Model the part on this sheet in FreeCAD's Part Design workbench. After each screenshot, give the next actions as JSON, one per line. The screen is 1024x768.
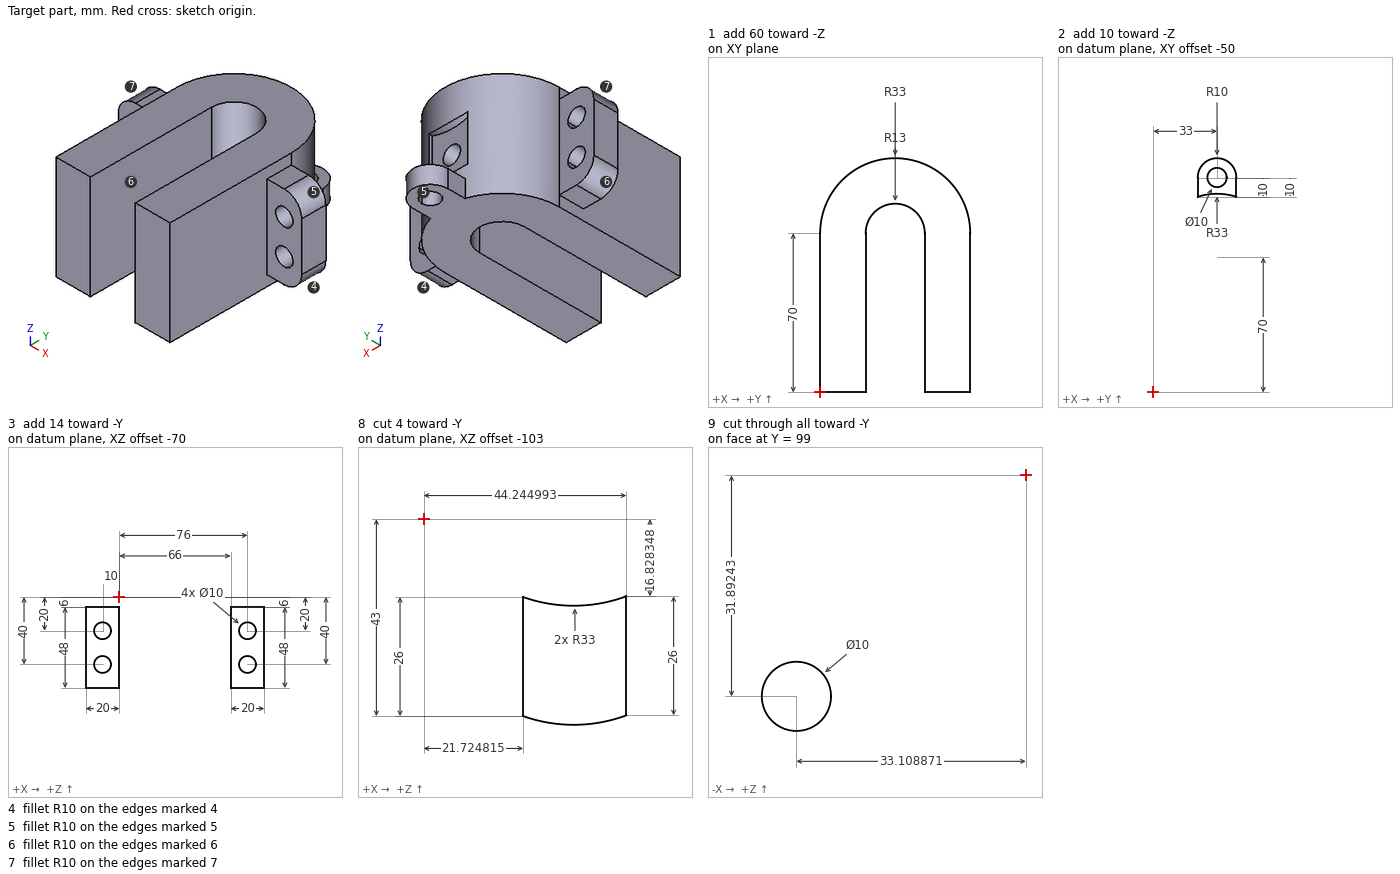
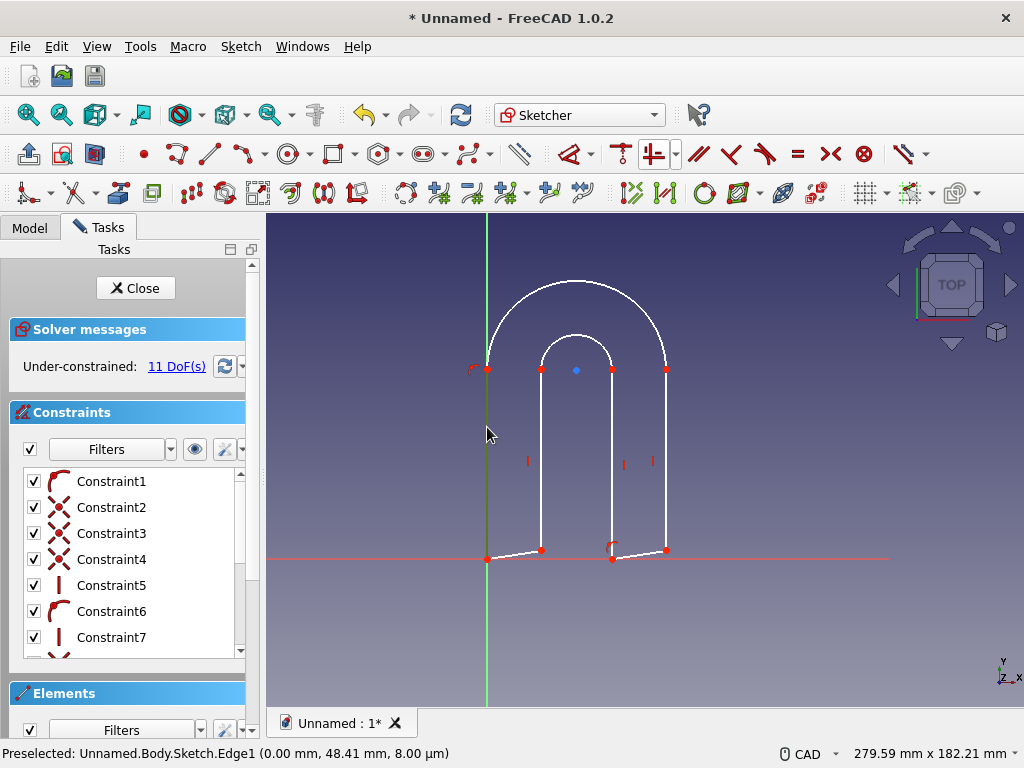
{"action": "left_click", "coordinate": [629, 298]}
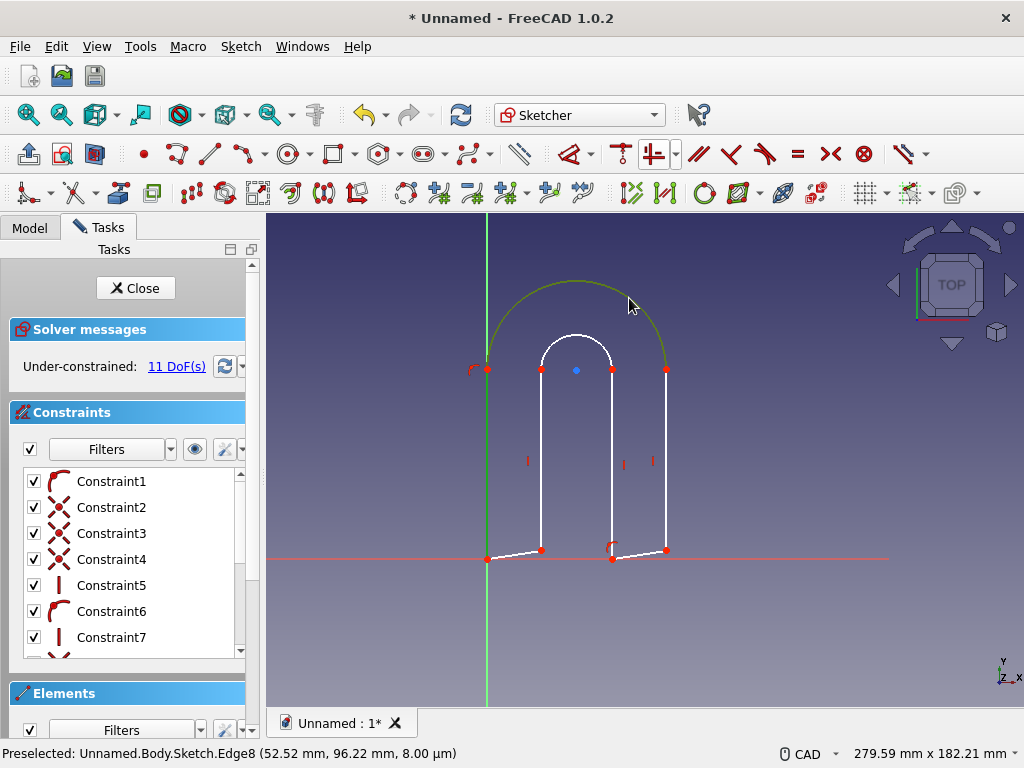
{"action": "key", "text": "t"}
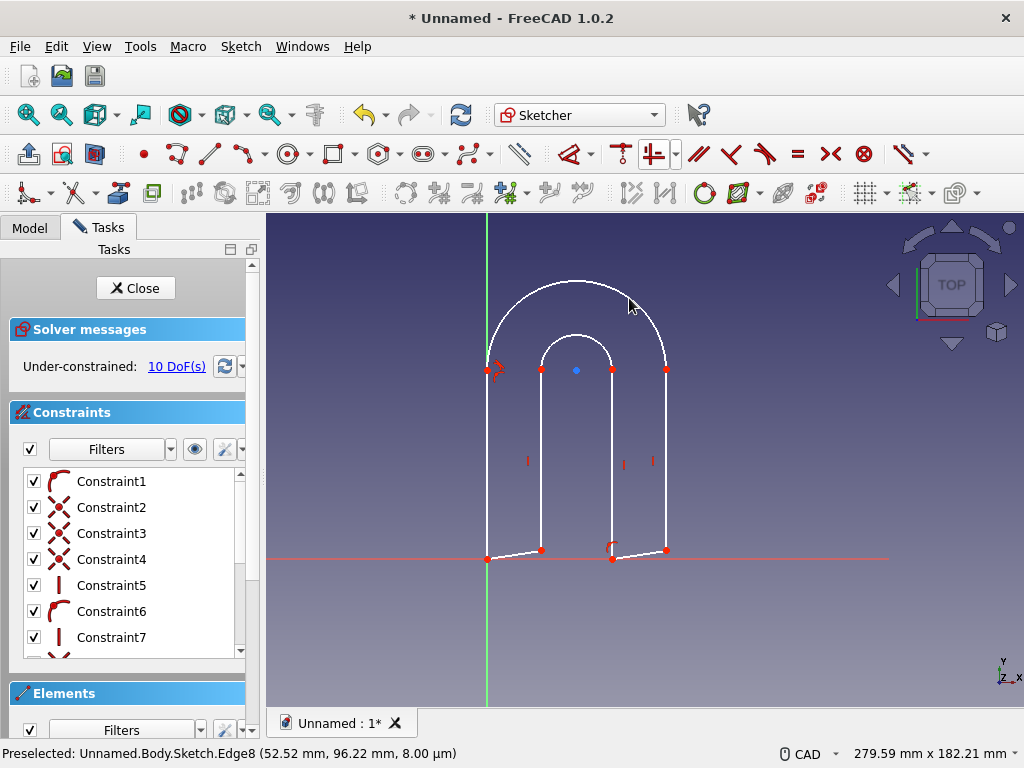
{"action": "left_click", "coordinate": [541, 497]}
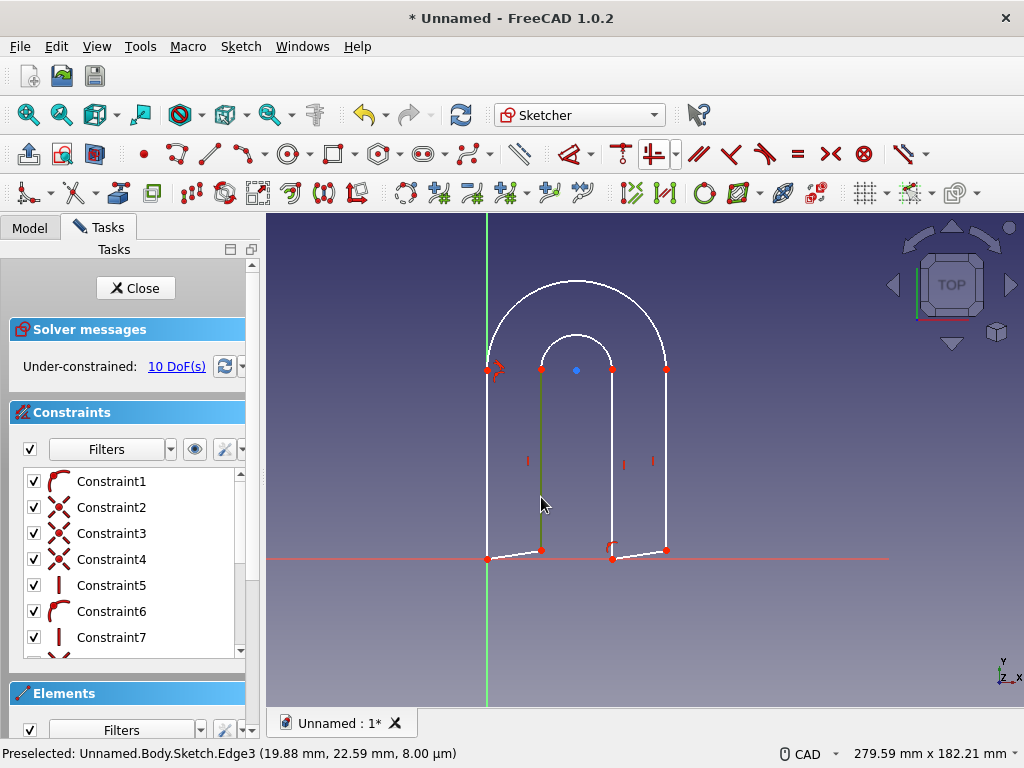
{"action": "left_click", "coordinate": [597, 342]}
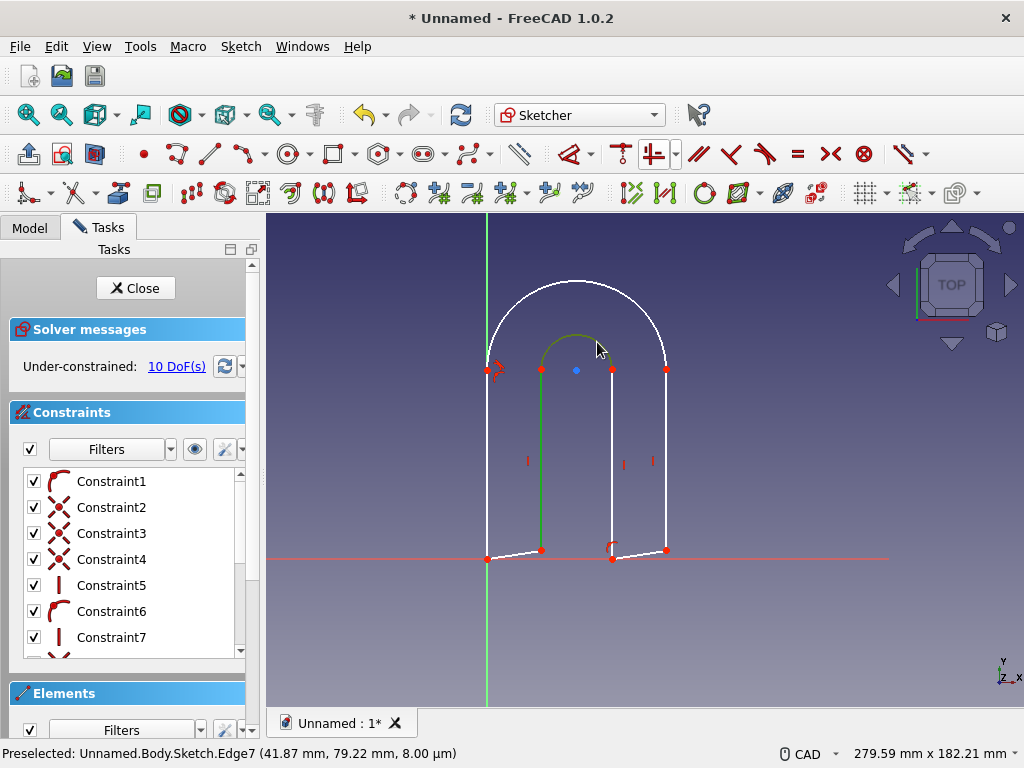
{"action": "left_click", "coordinate": [765, 154]}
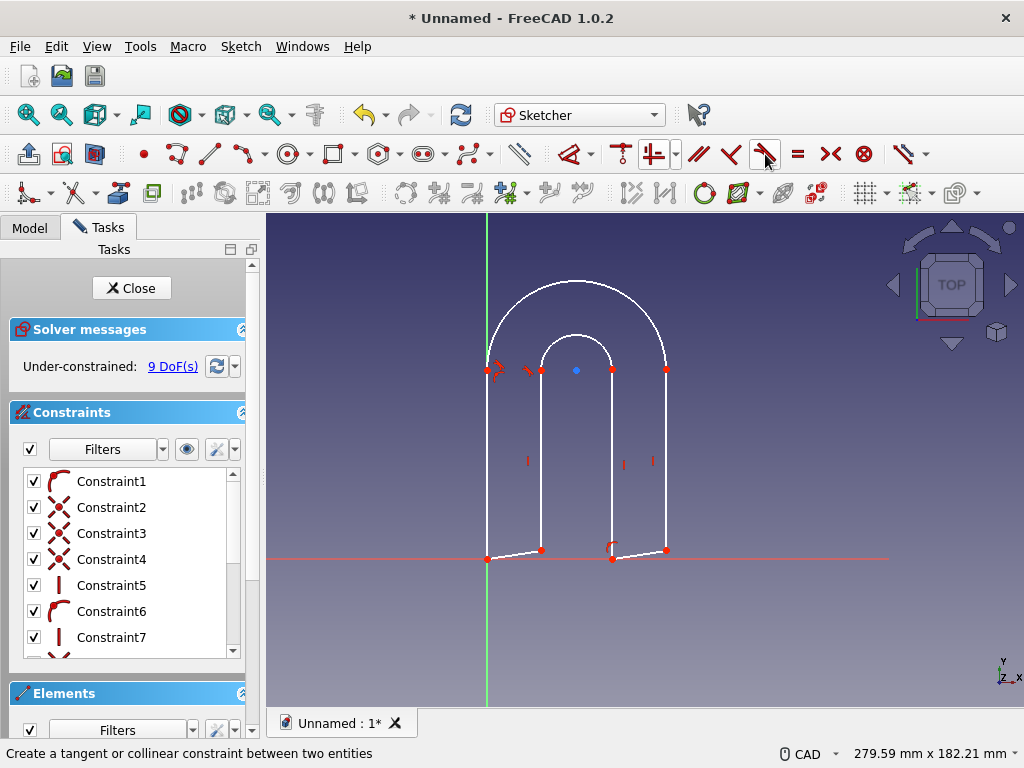
{"action": "left_click", "coordinate": [612, 427]}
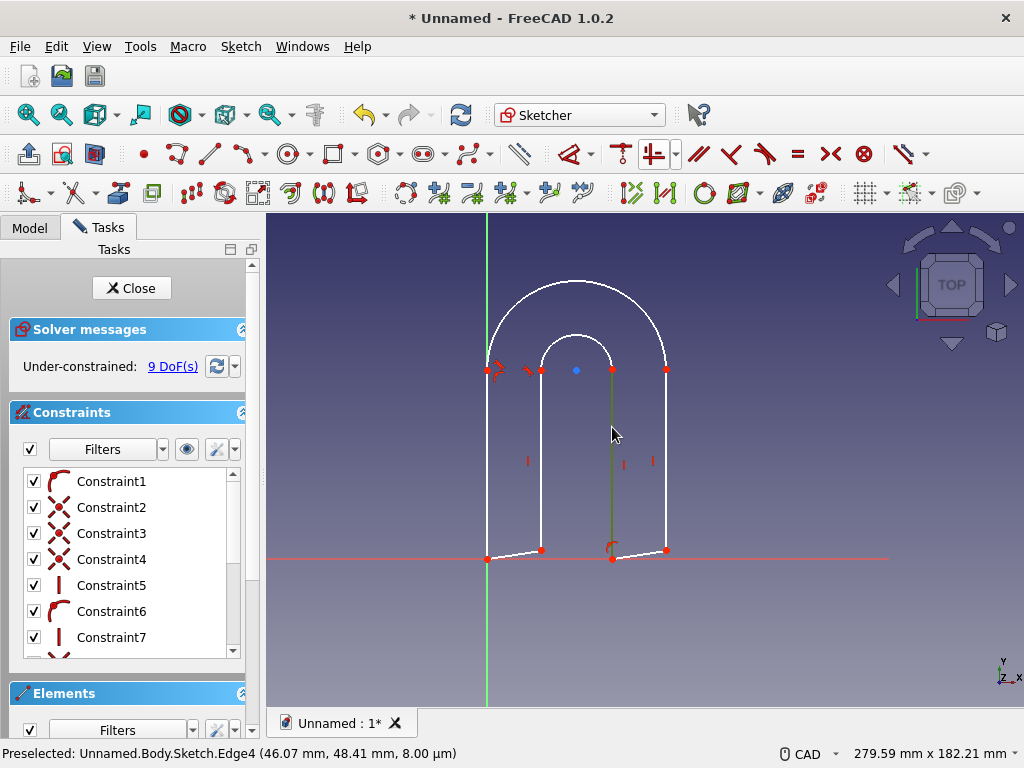
{"action": "left_click", "coordinate": [597, 342]}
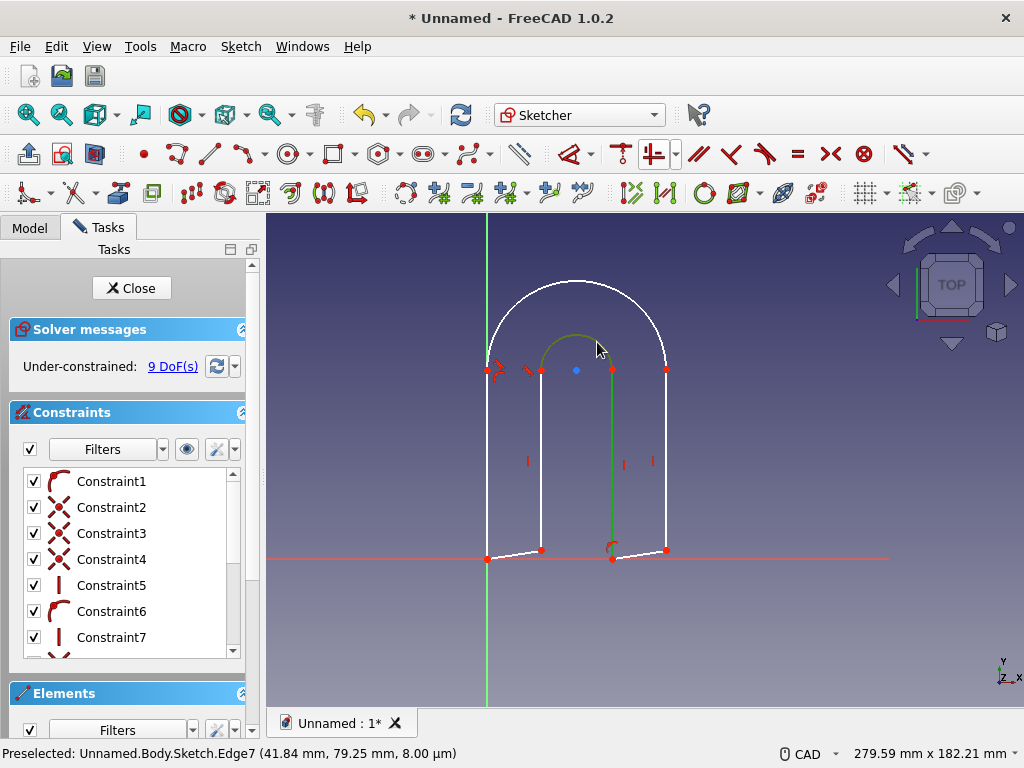
{"action": "key", "text": "t"}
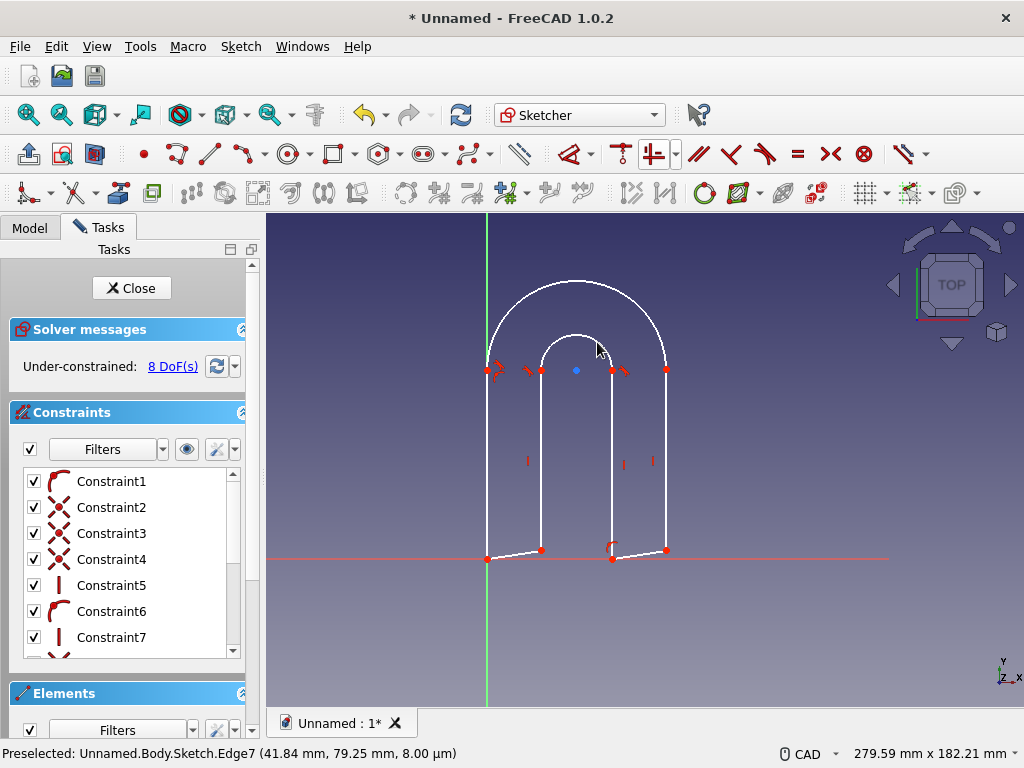
{"action": "left_click", "coordinate": [666, 497]}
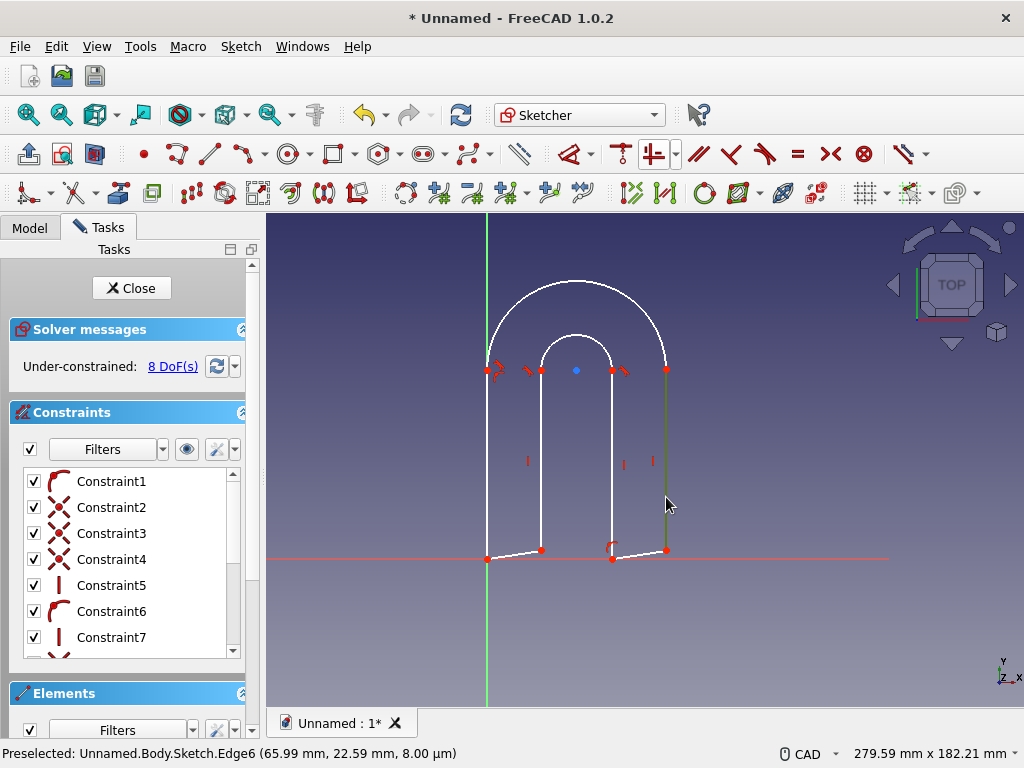
{"action": "left_click", "coordinate": [629, 298]}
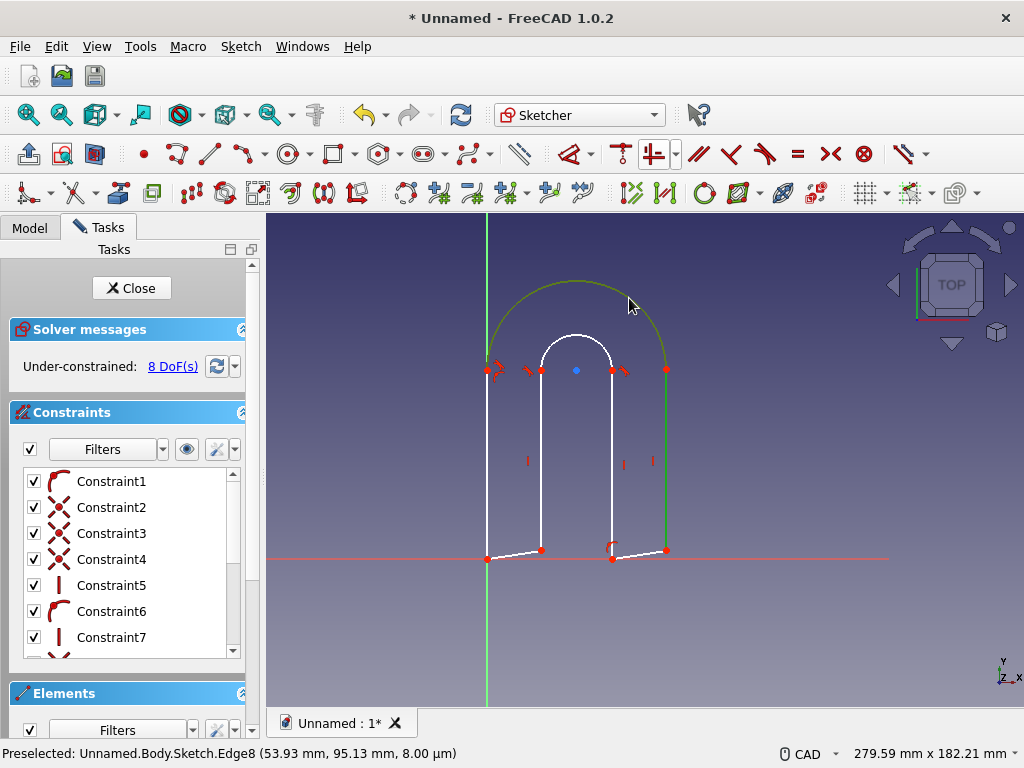
{"action": "left_click", "coordinate": [765, 154]}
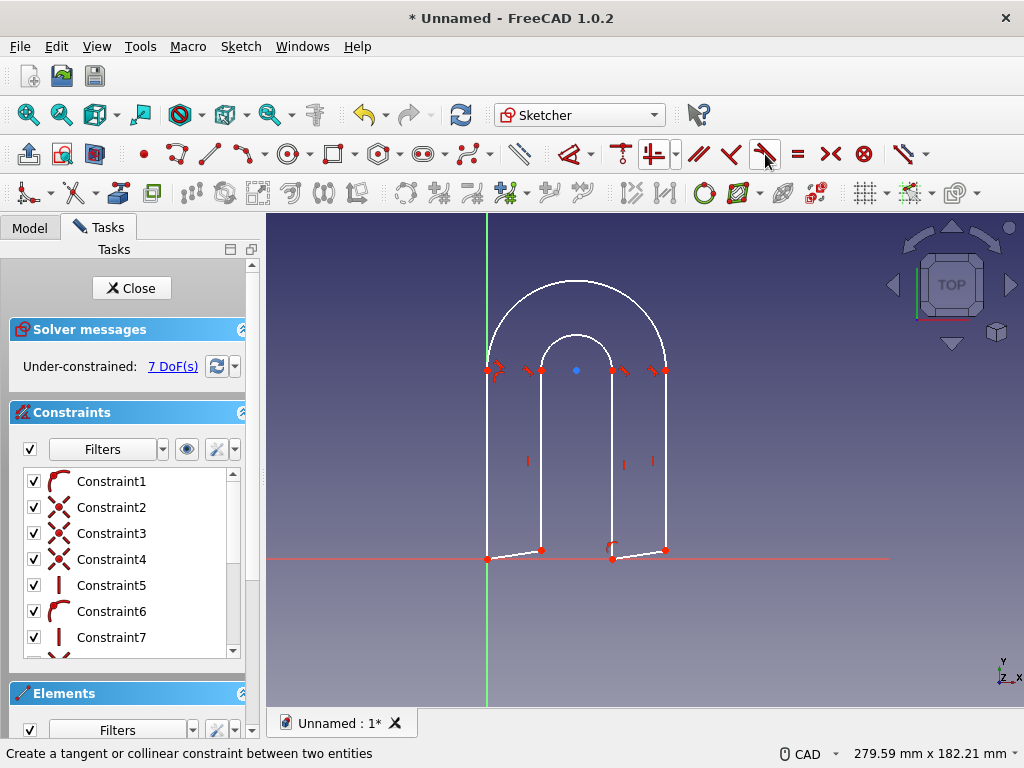
{"action": "left_click", "coordinate": [503, 557]}